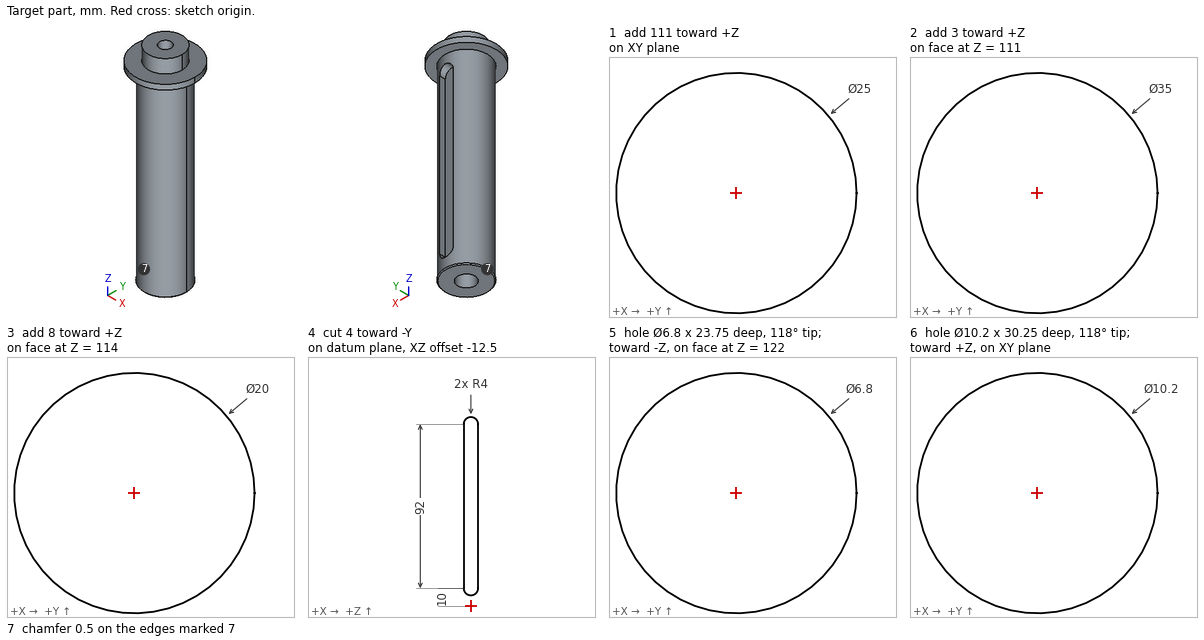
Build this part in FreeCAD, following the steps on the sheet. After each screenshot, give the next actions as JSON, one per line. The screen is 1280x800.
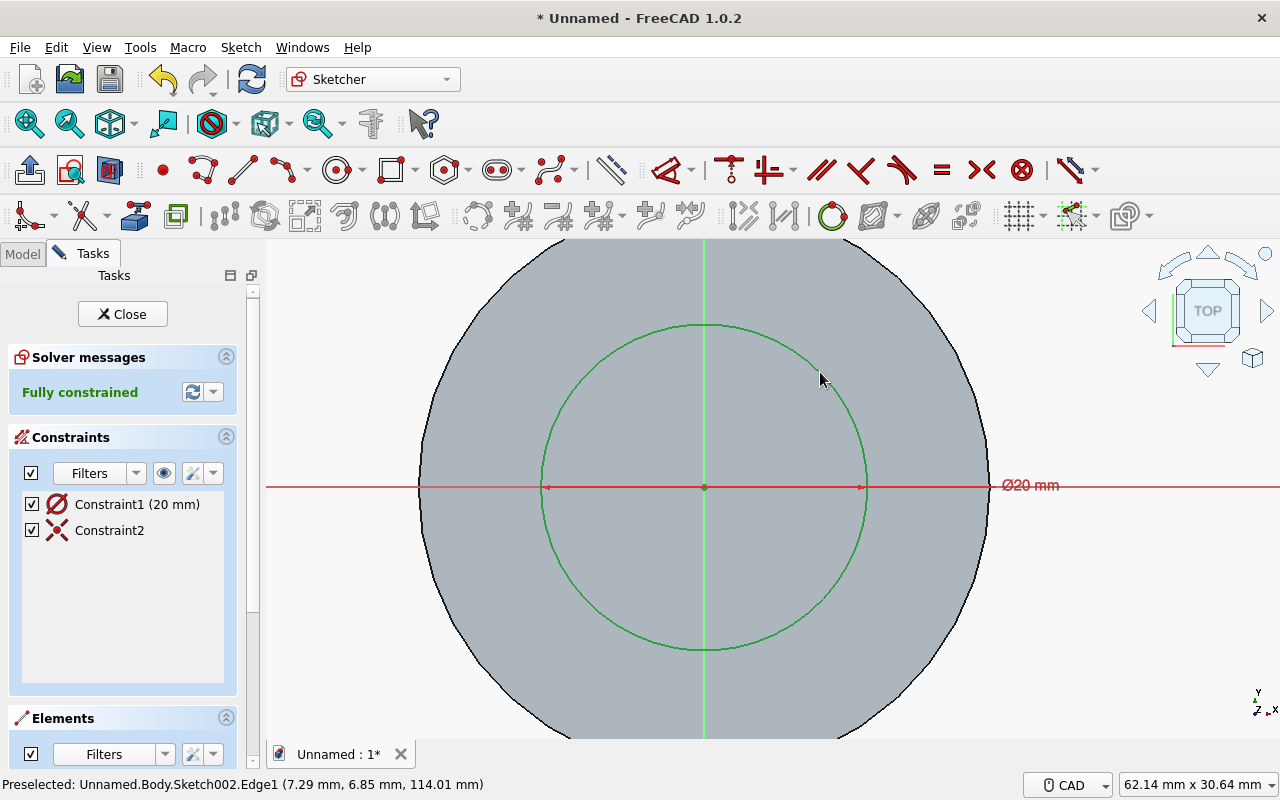
{"action": "left_click", "coordinate": [123, 314]}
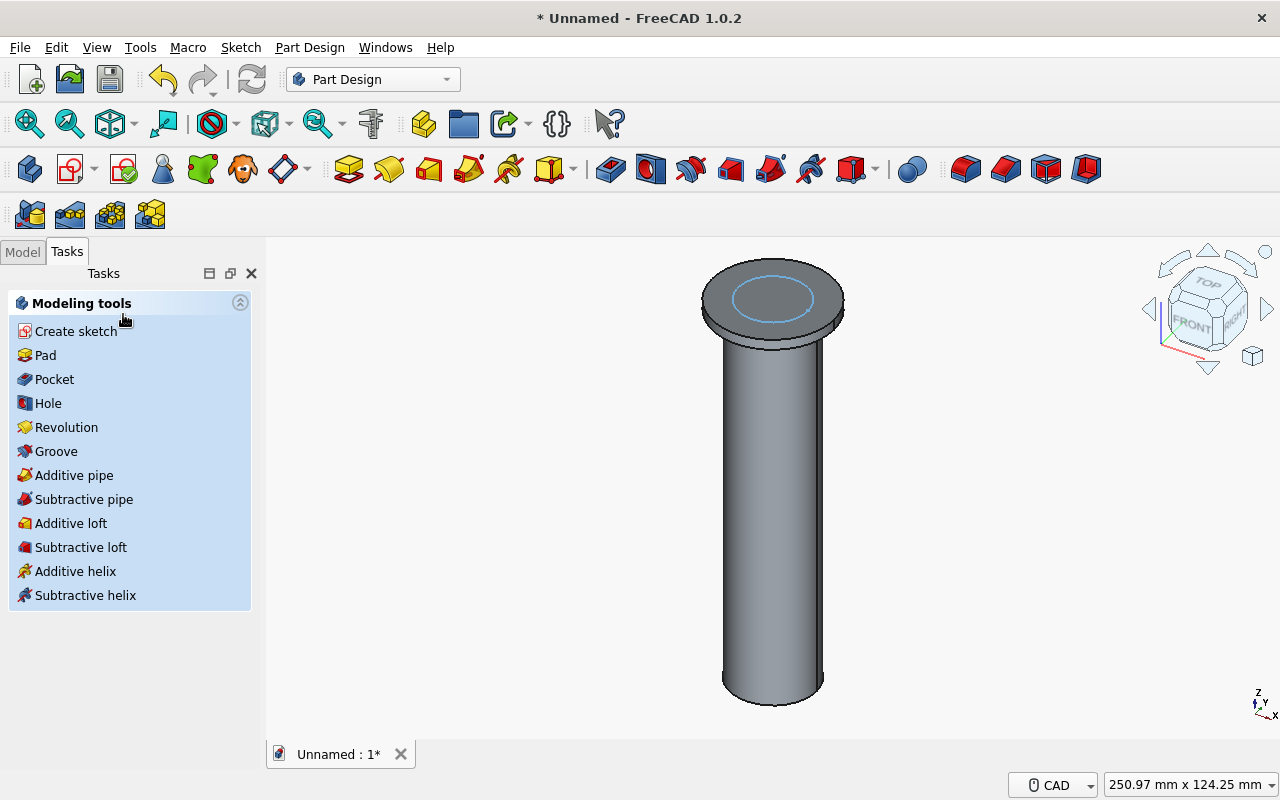
{"action": "left_click", "coordinate": [350, 170]}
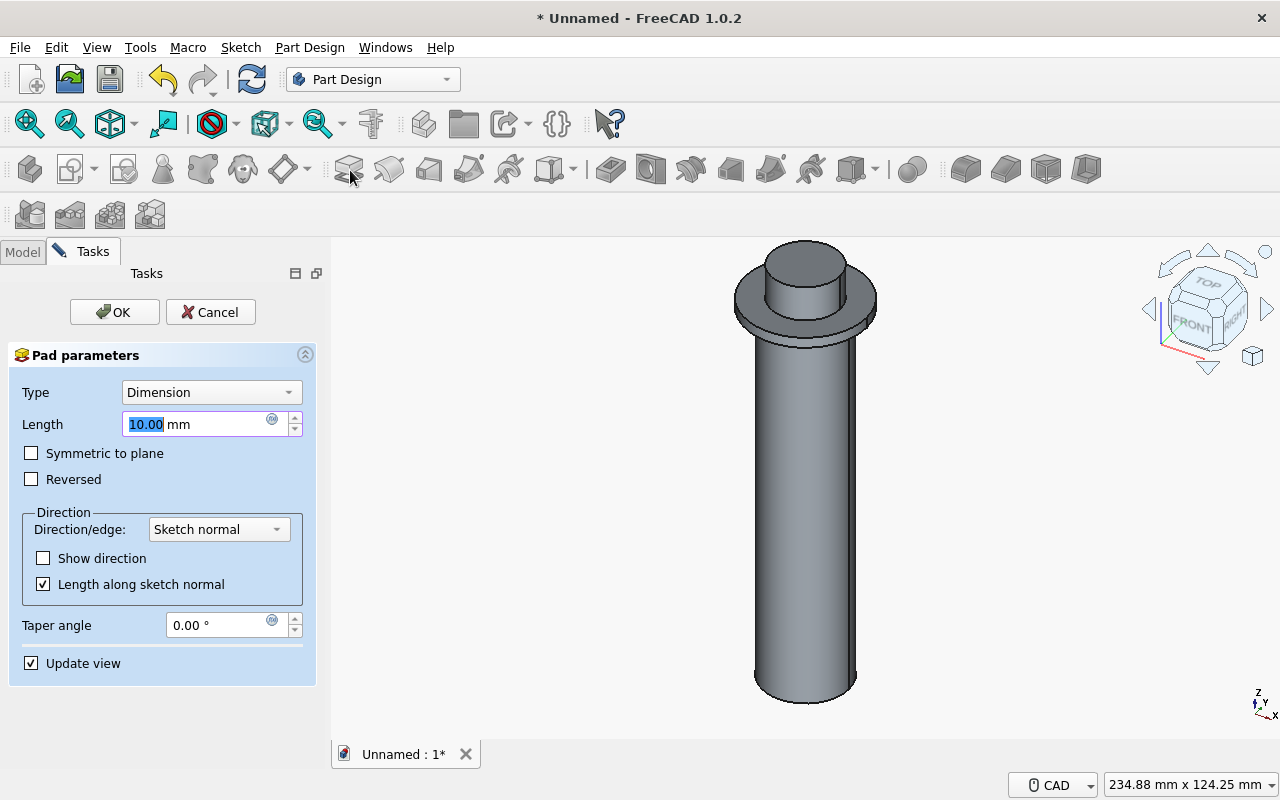
{"action": "type", "text": "8"}
{"action": "key", "text": "Tab"}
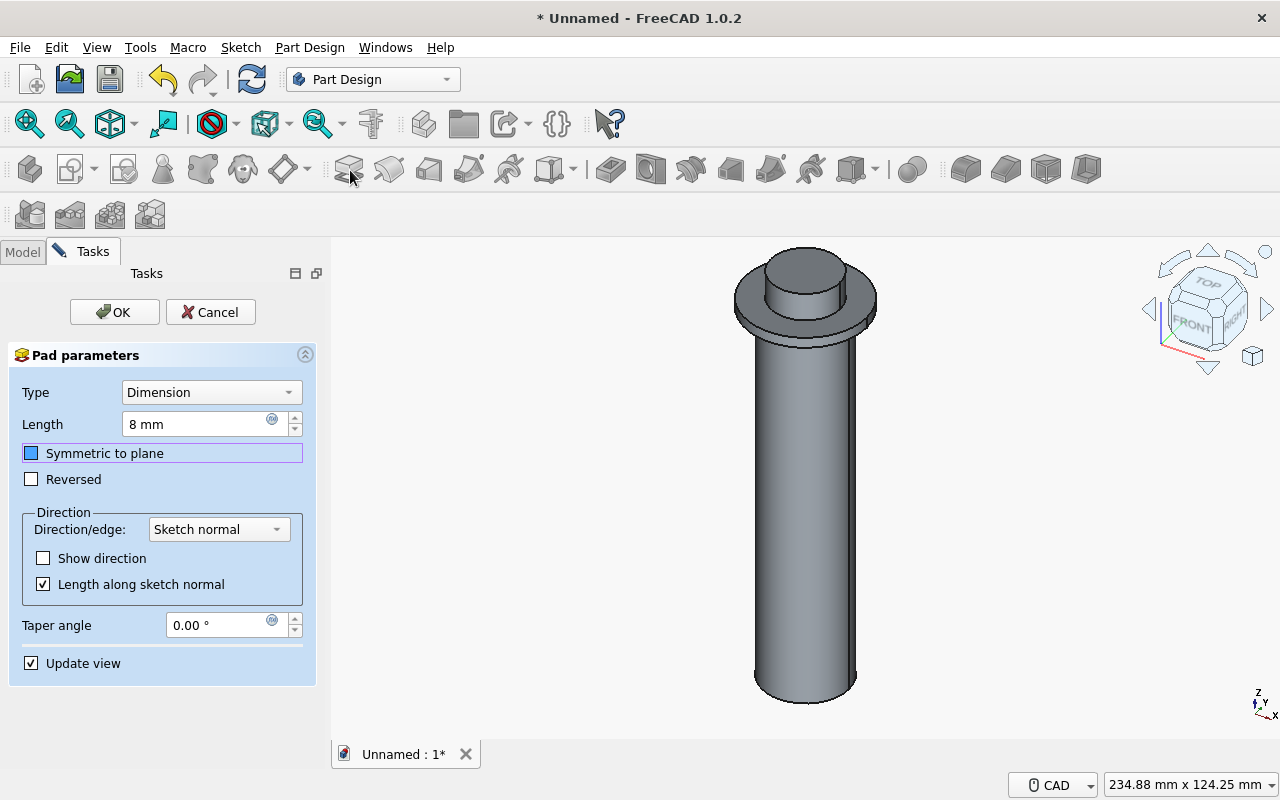
{"action": "left_click", "coordinate": [115, 312]}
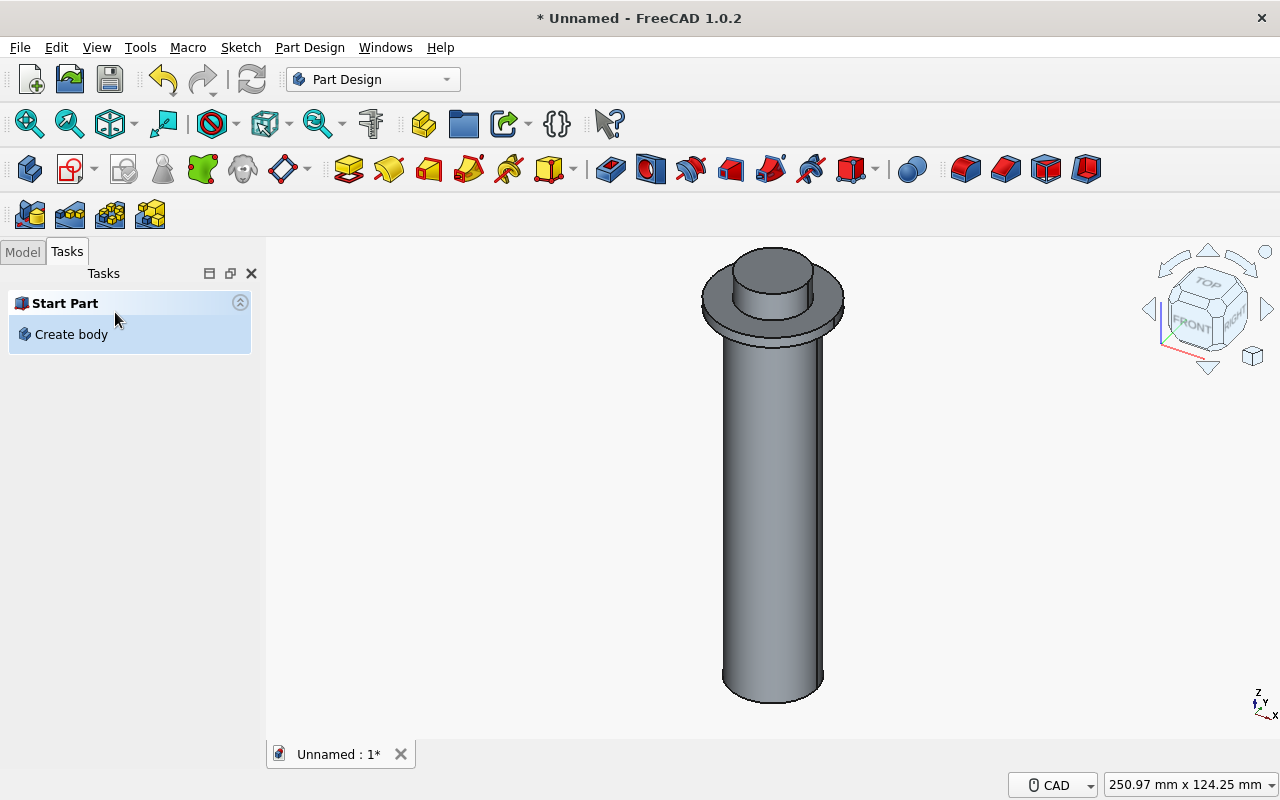
{"action": "left_click", "coordinate": [30, 124]}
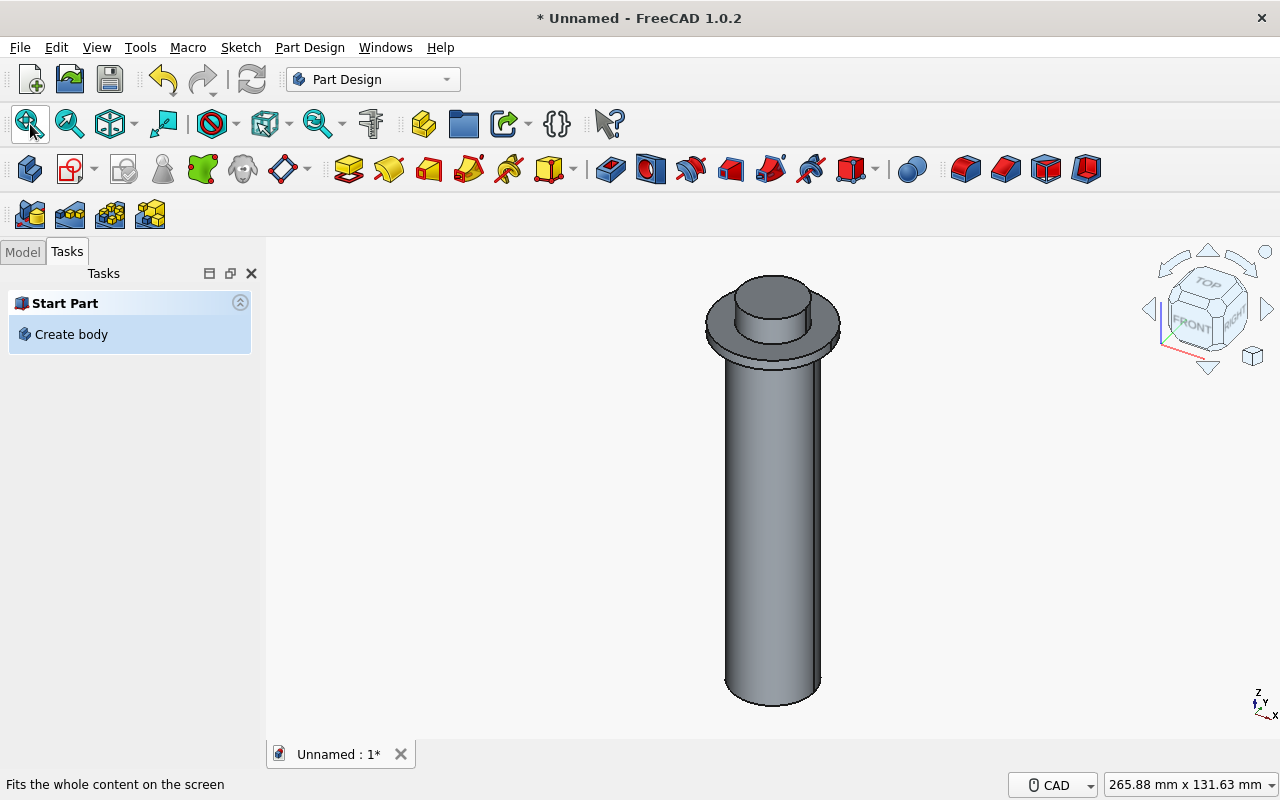
{"action": "left_click", "coordinate": [23, 251]}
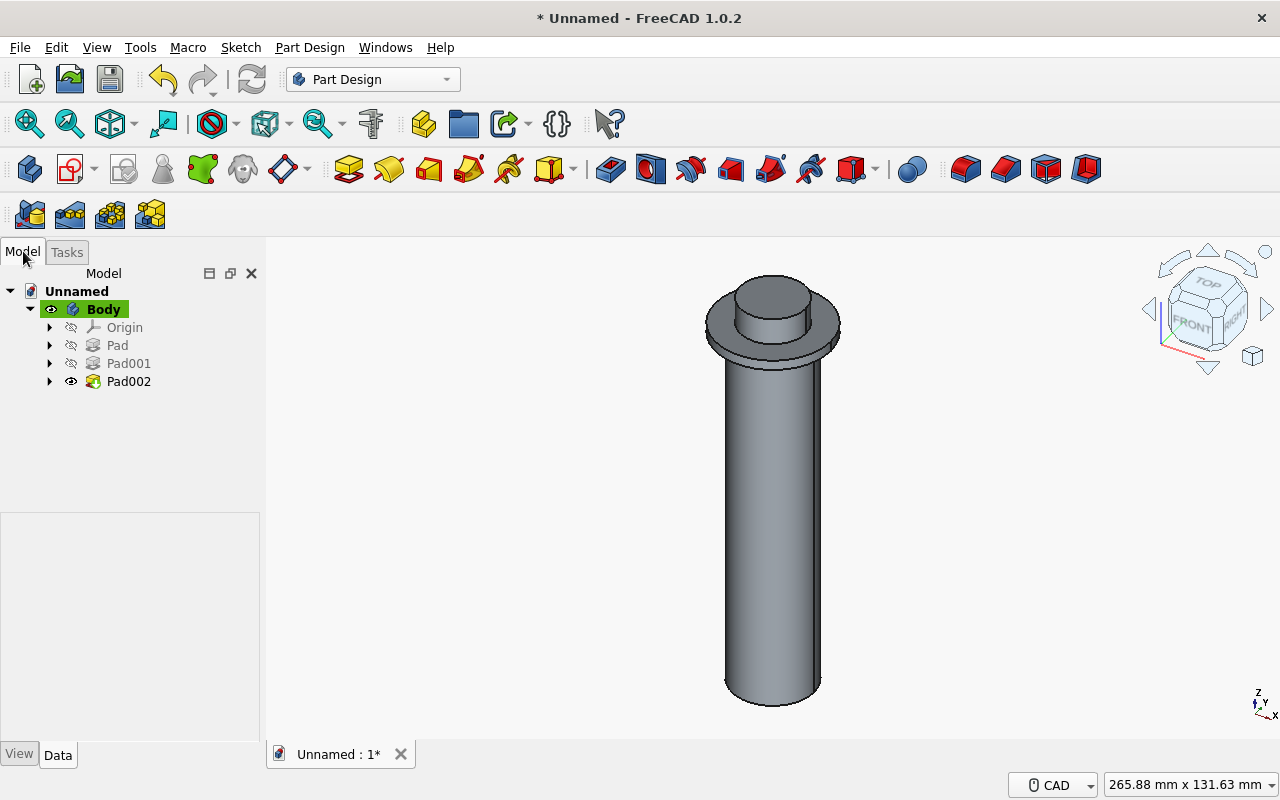
{"action": "left_click", "coordinate": [50, 327]}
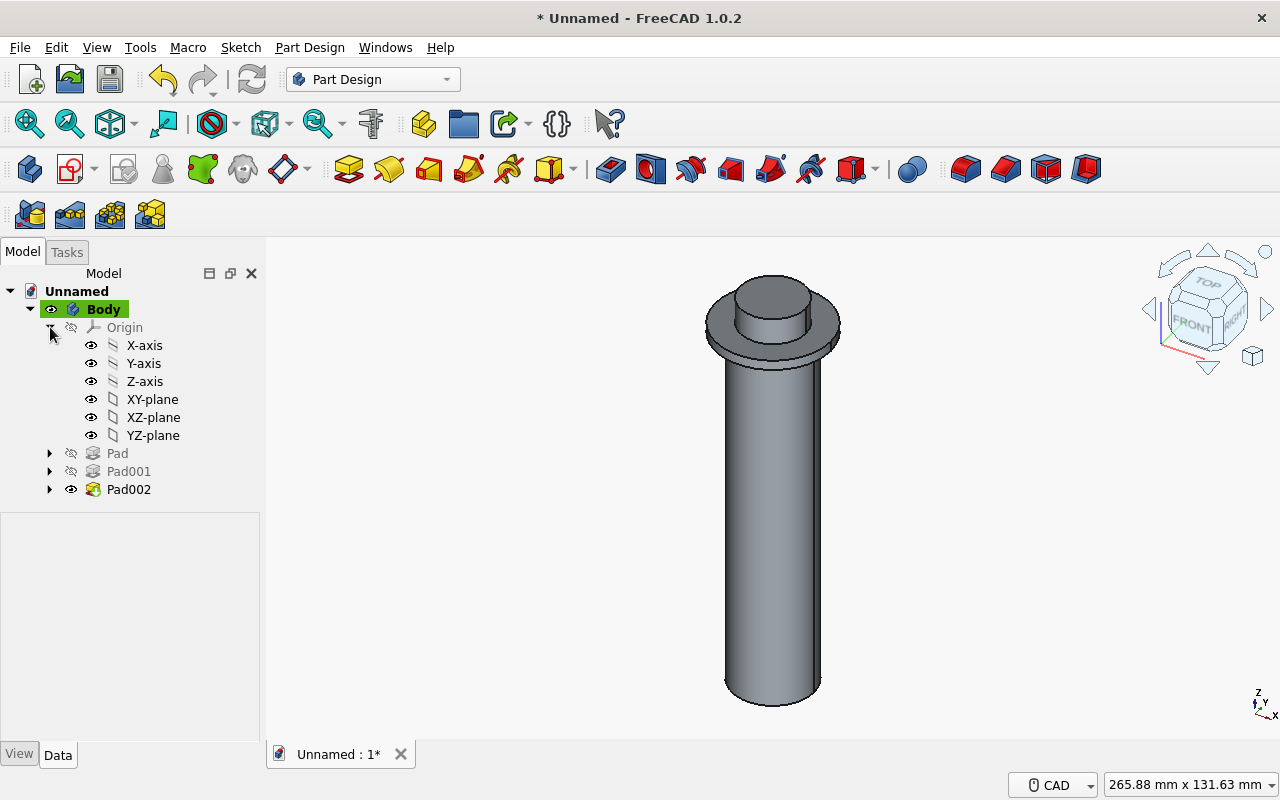
{"action": "left_click", "coordinate": [136, 417]}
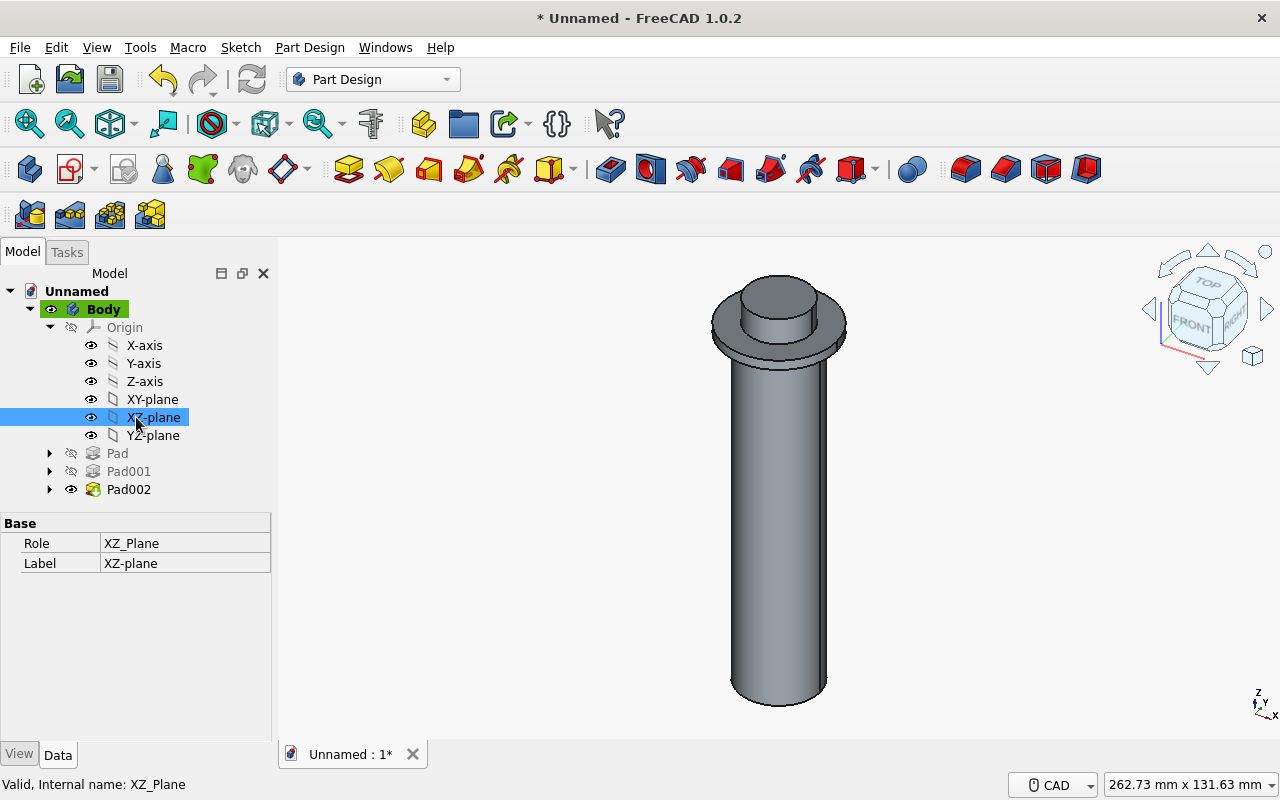
{"action": "left_click", "coordinate": [284, 170]}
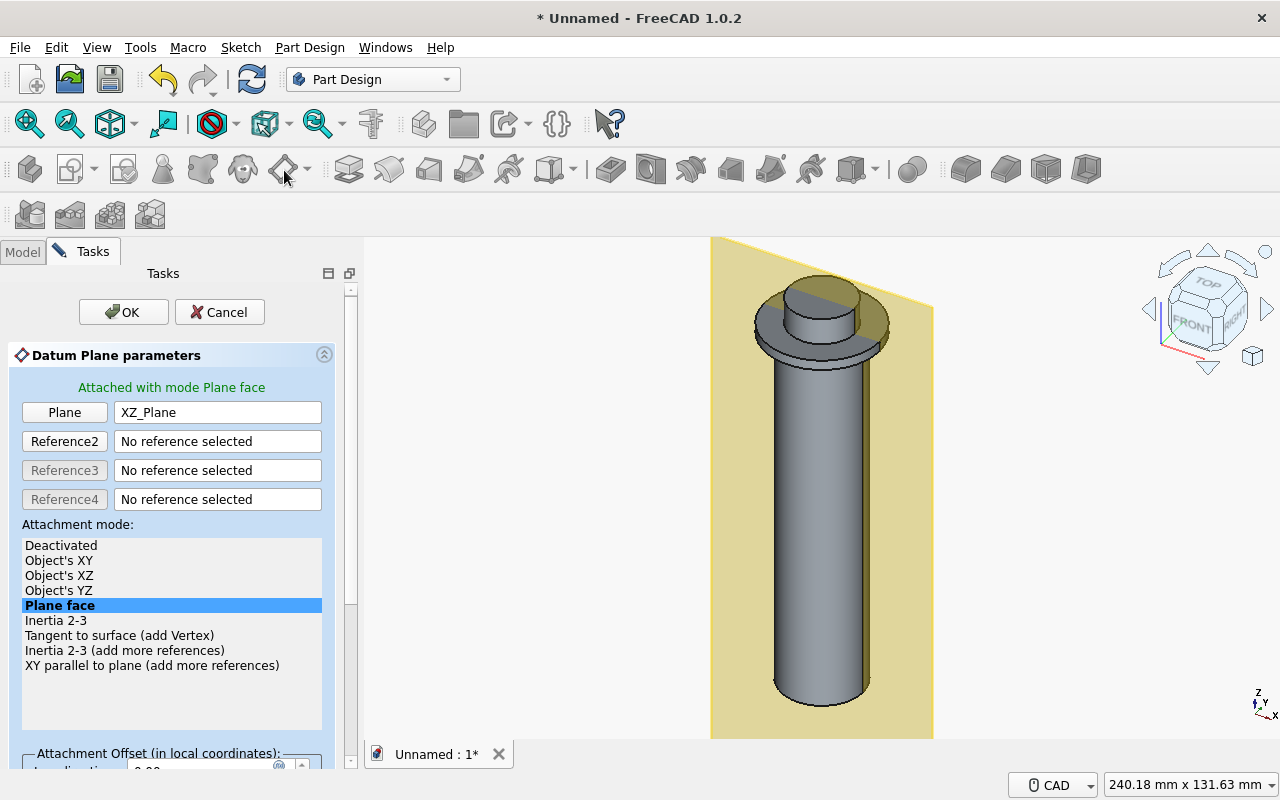
{"action": "scroll", "coordinate": [351, 526], "scroll_direction": "down", "scroll_amount": 3}